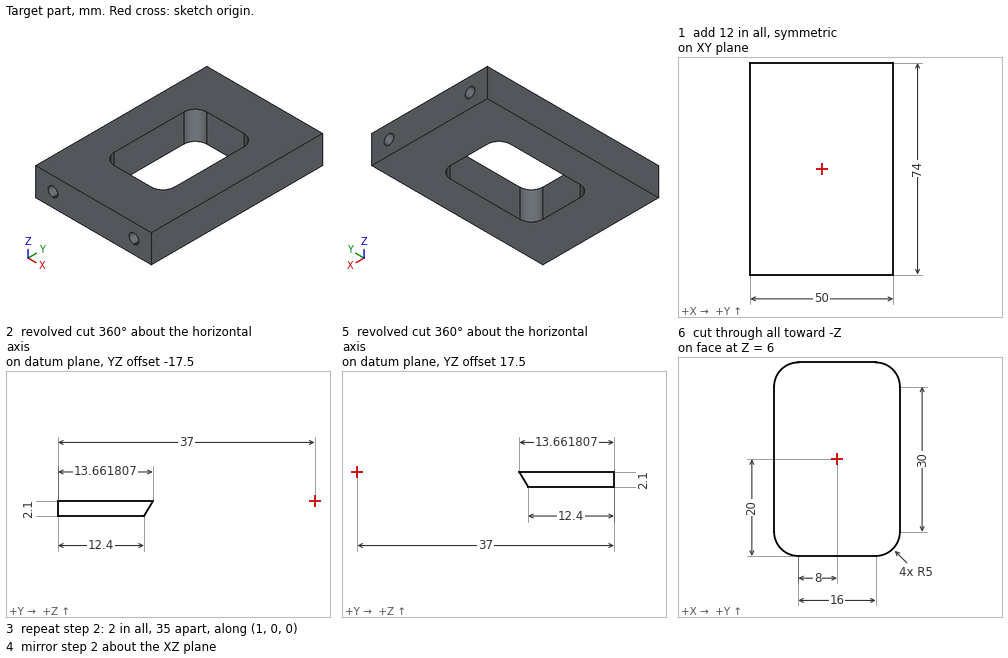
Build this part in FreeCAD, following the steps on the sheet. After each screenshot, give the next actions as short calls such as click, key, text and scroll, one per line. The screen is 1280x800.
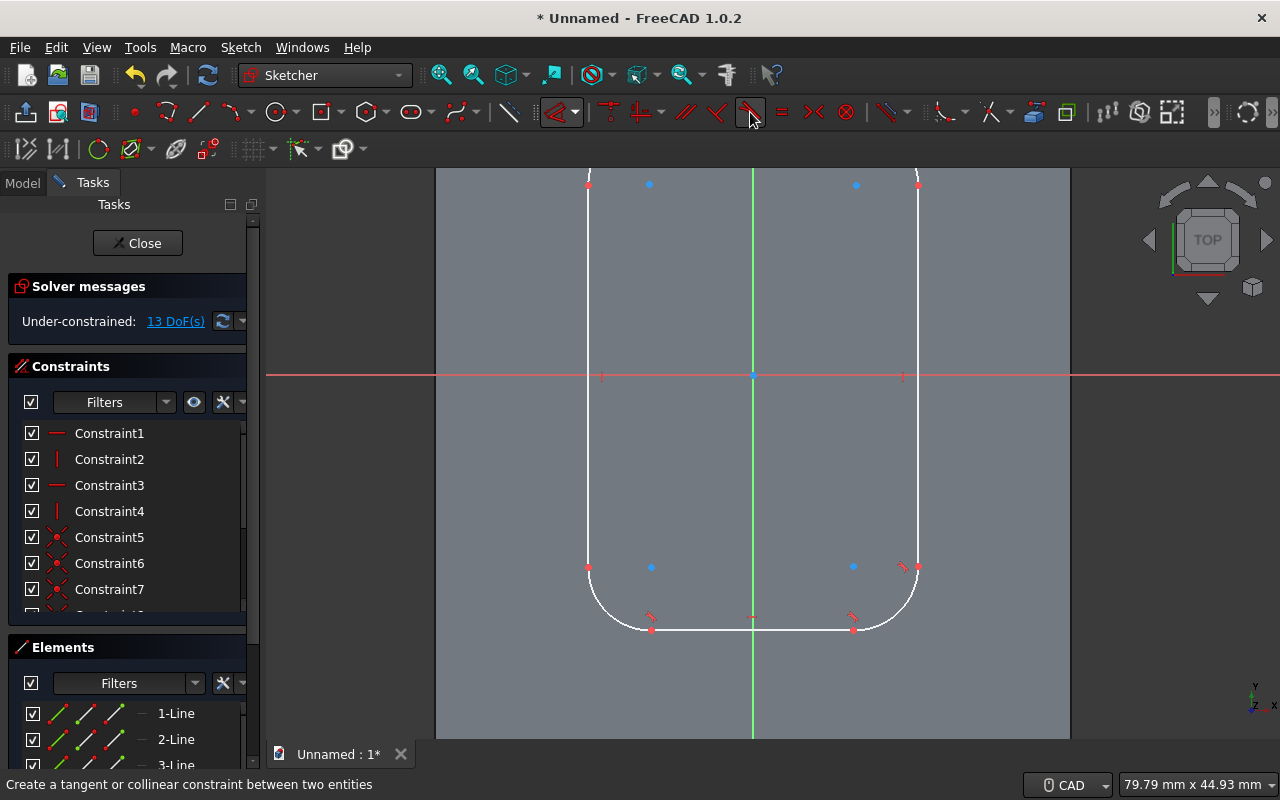
click(918, 452)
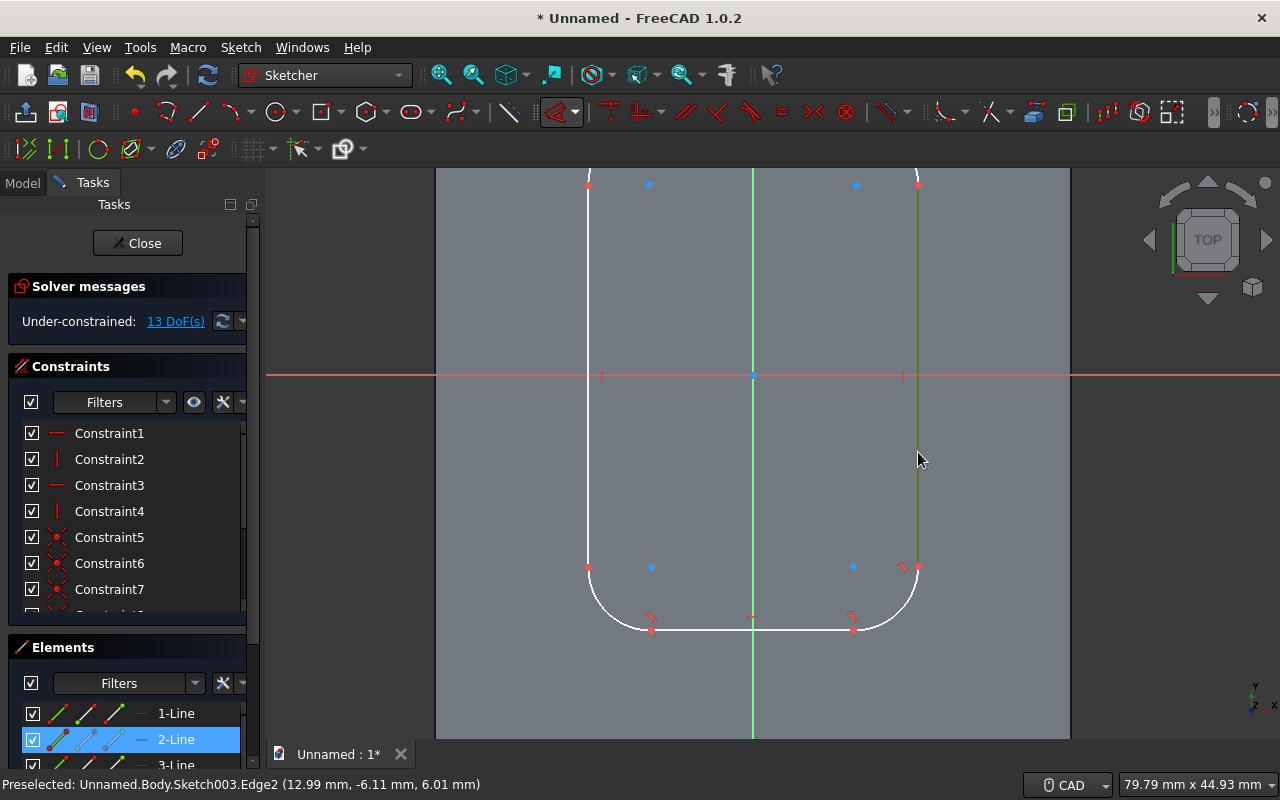
scroll(606, 612, down, 2)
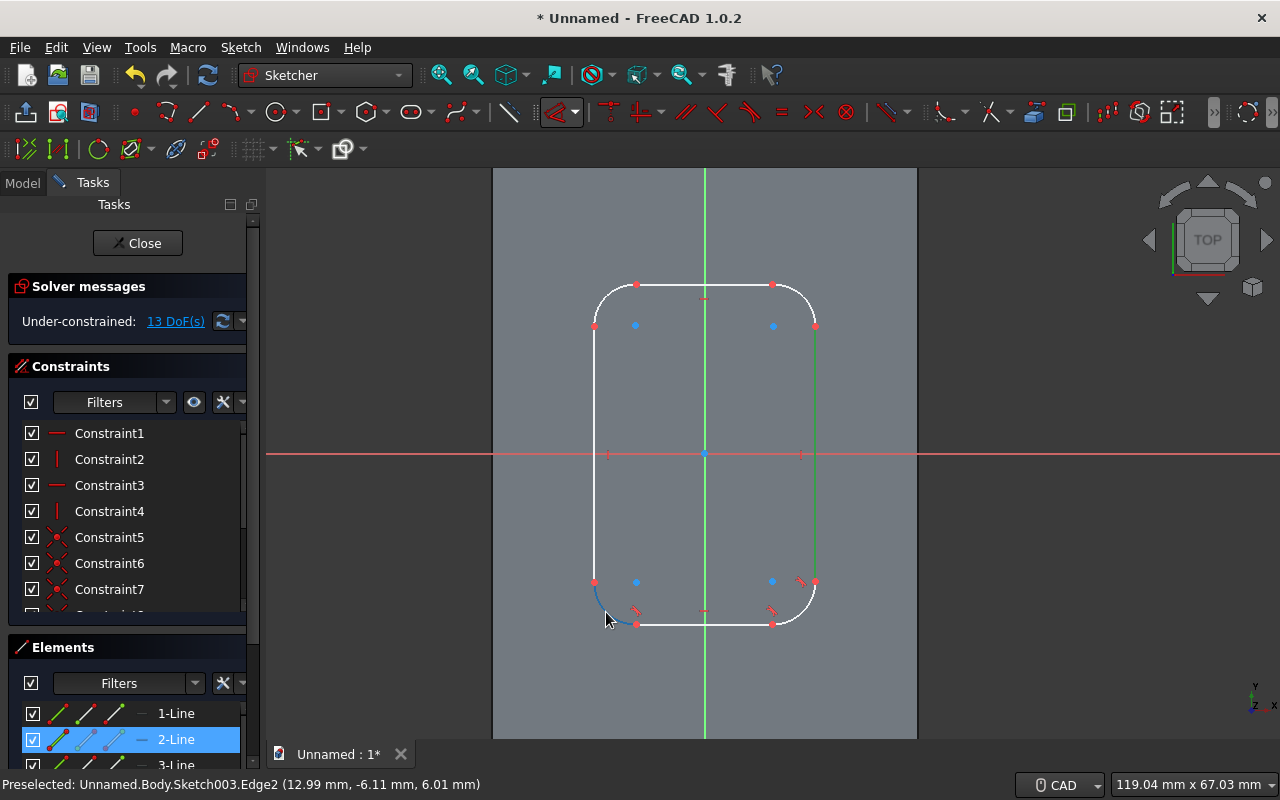
click(811, 307)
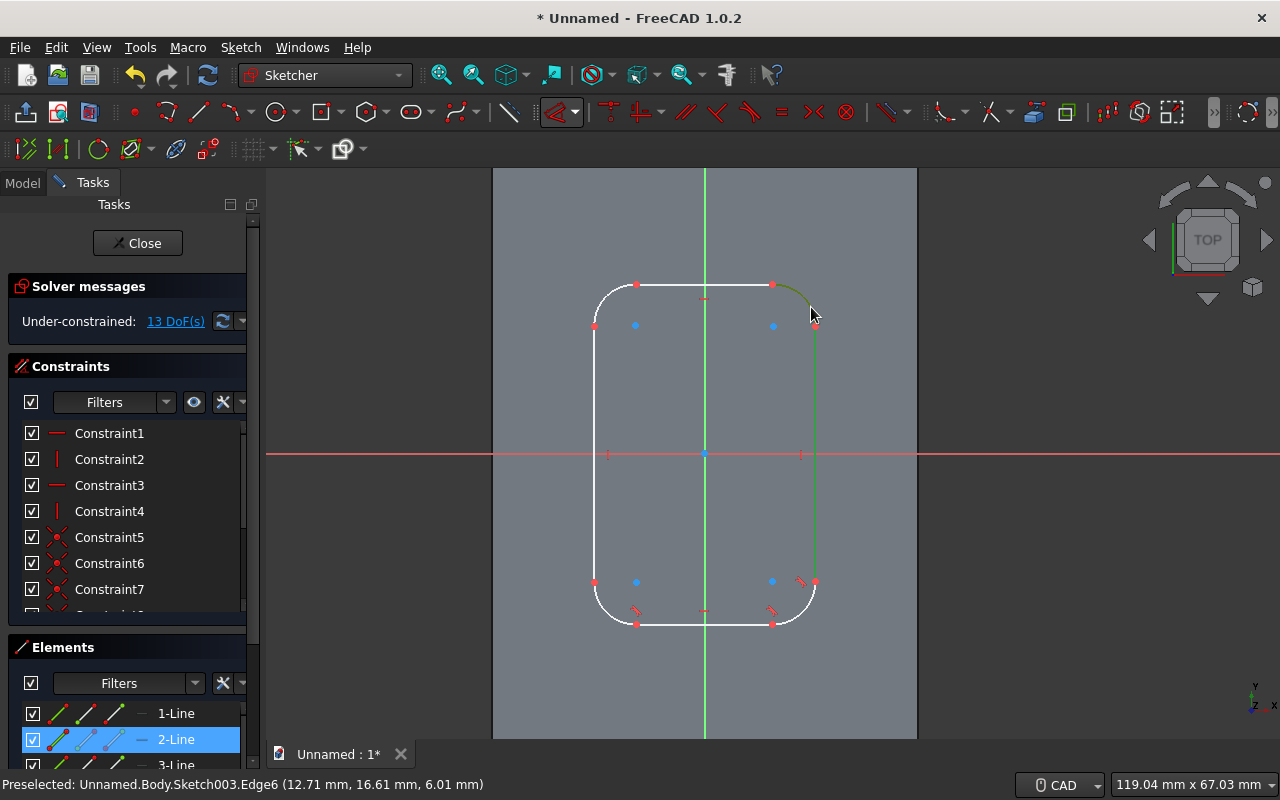
click(750, 112)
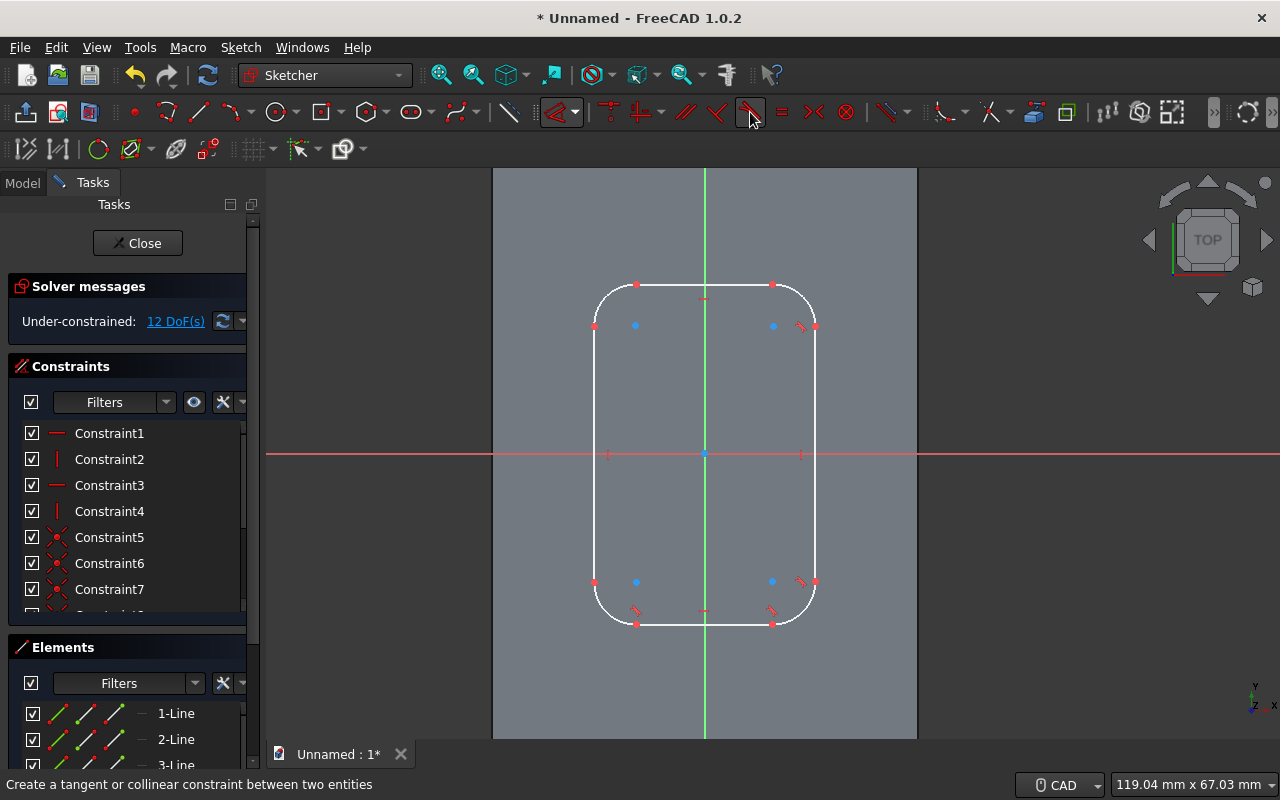
click(732, 285)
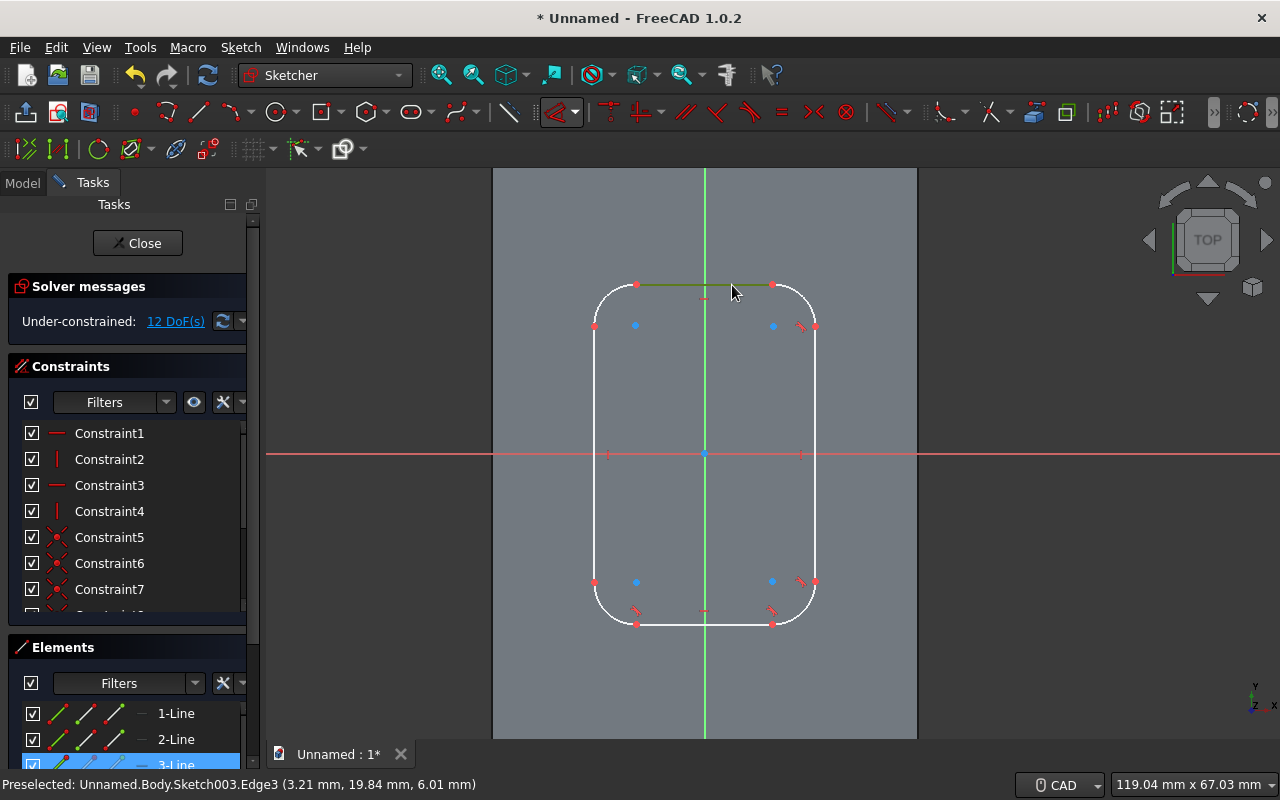
click(811, 307)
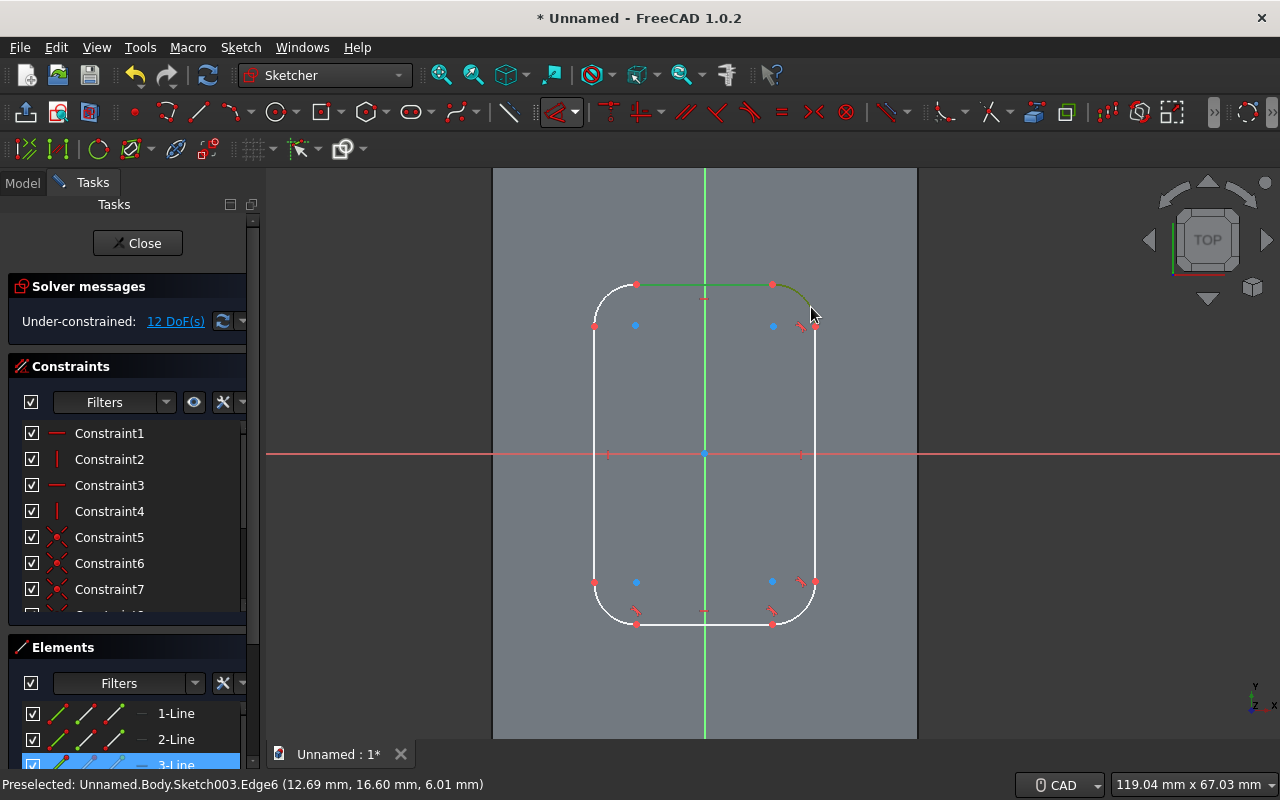
click(750, 112)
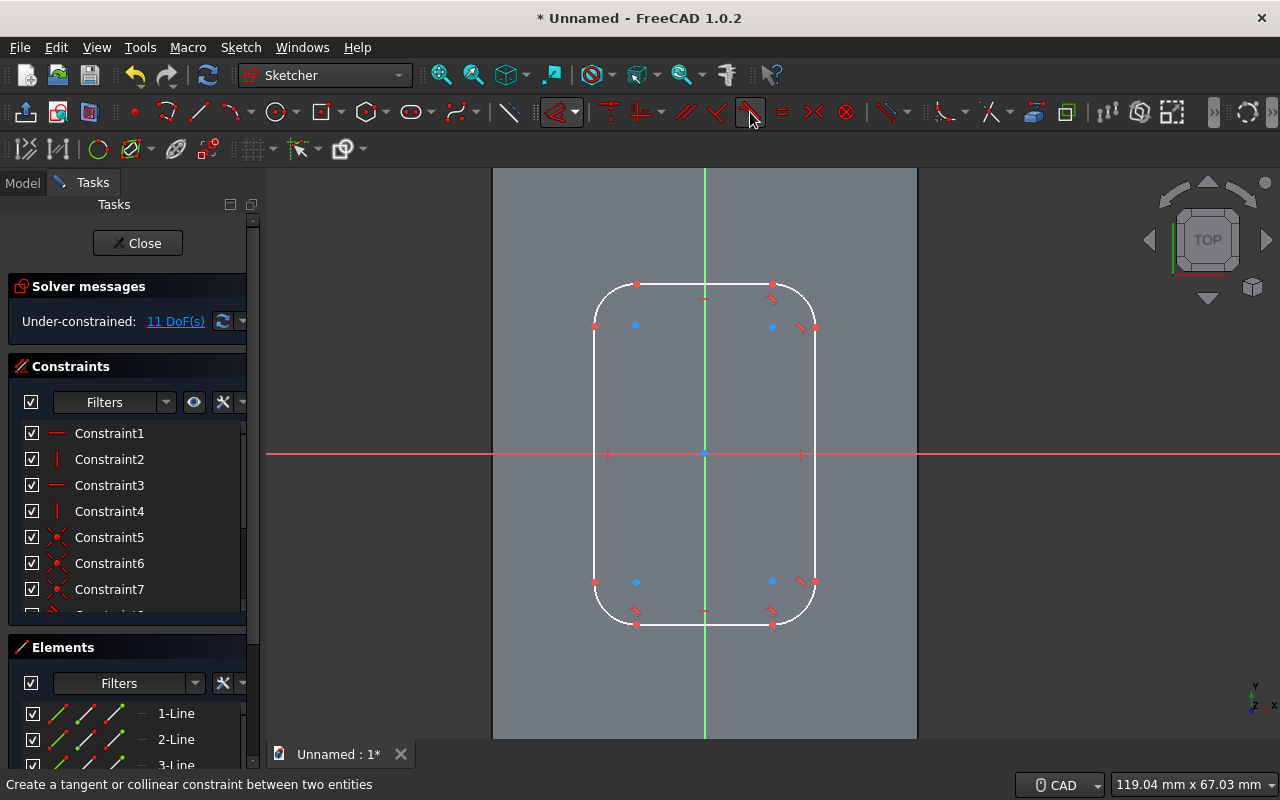
click(732, 284)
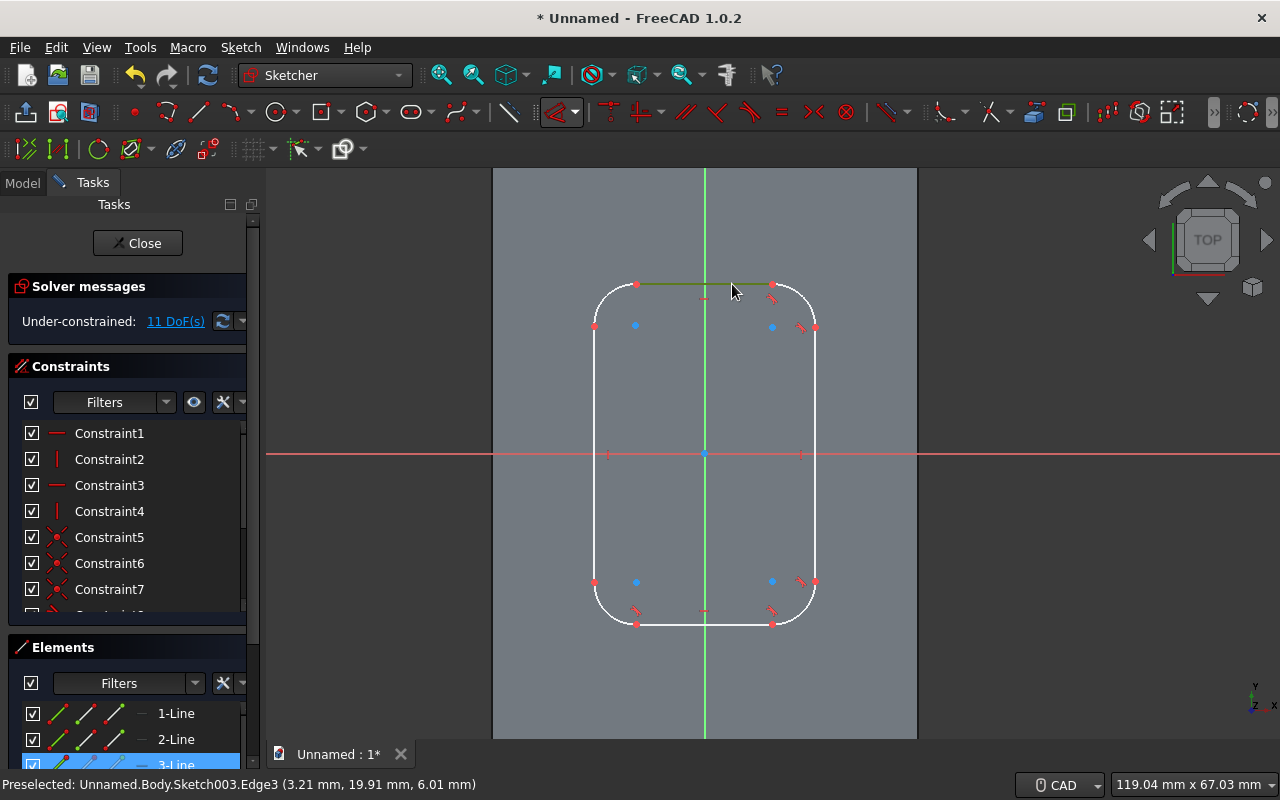
click(617, 289)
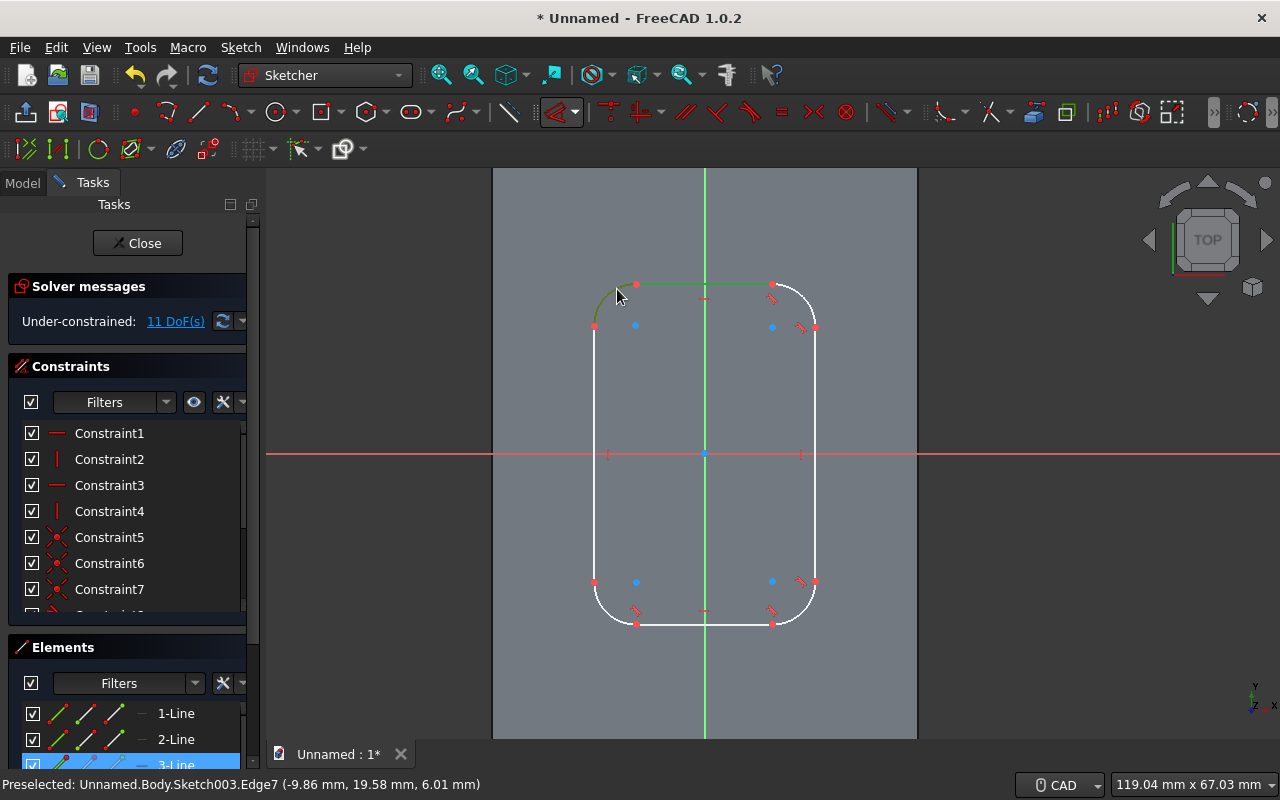
click(750, 112)